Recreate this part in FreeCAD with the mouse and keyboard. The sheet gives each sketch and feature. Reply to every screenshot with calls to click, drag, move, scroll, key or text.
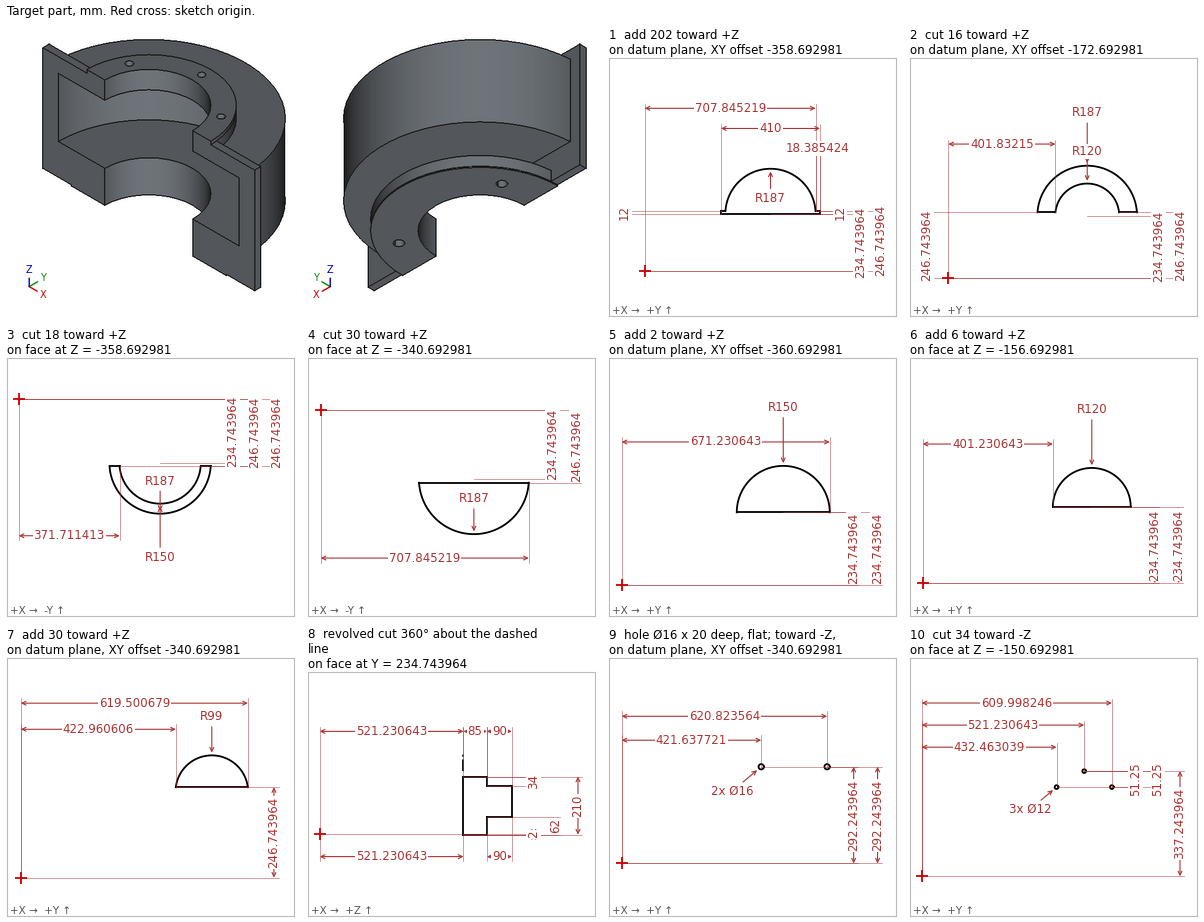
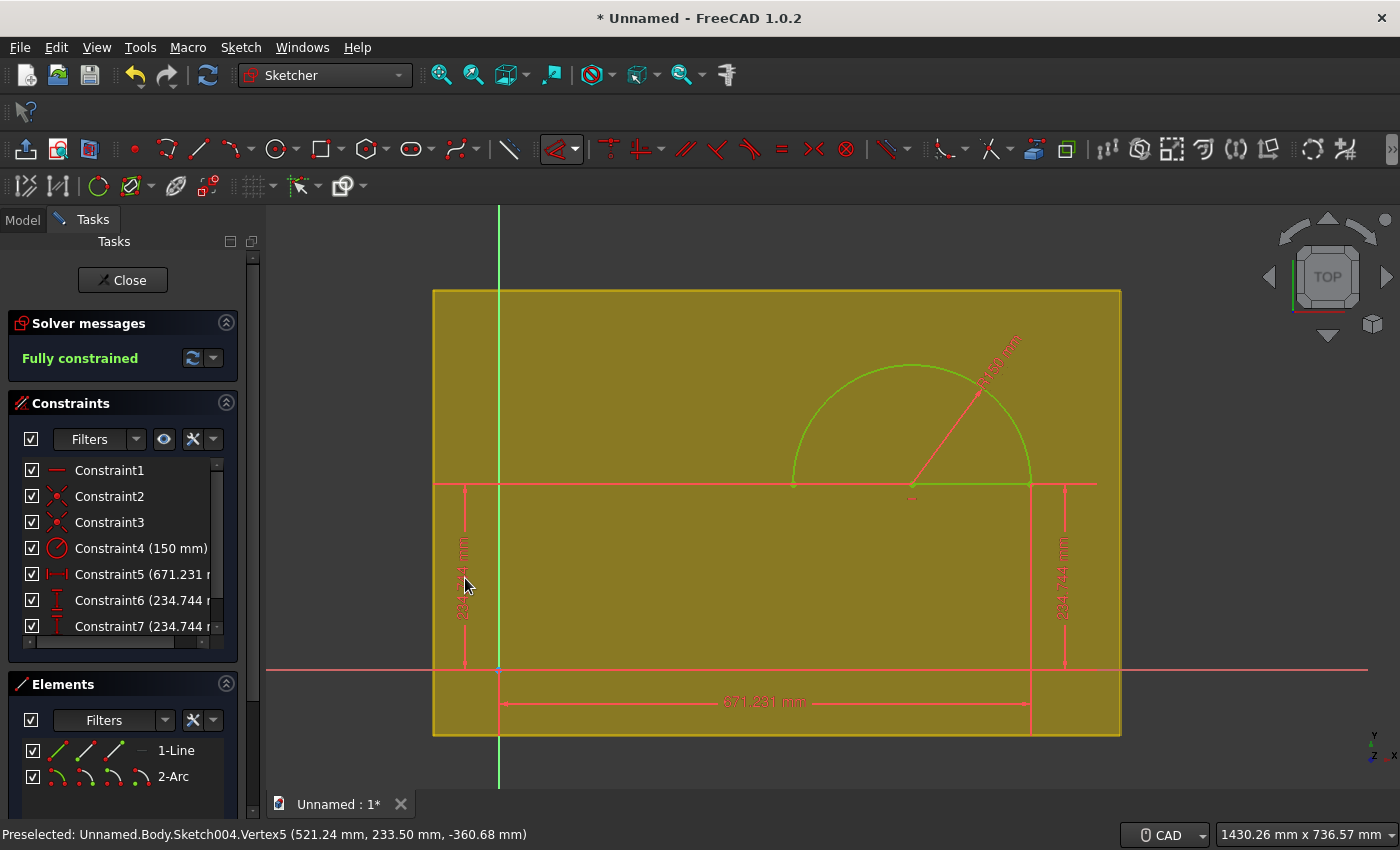
click(123, 280)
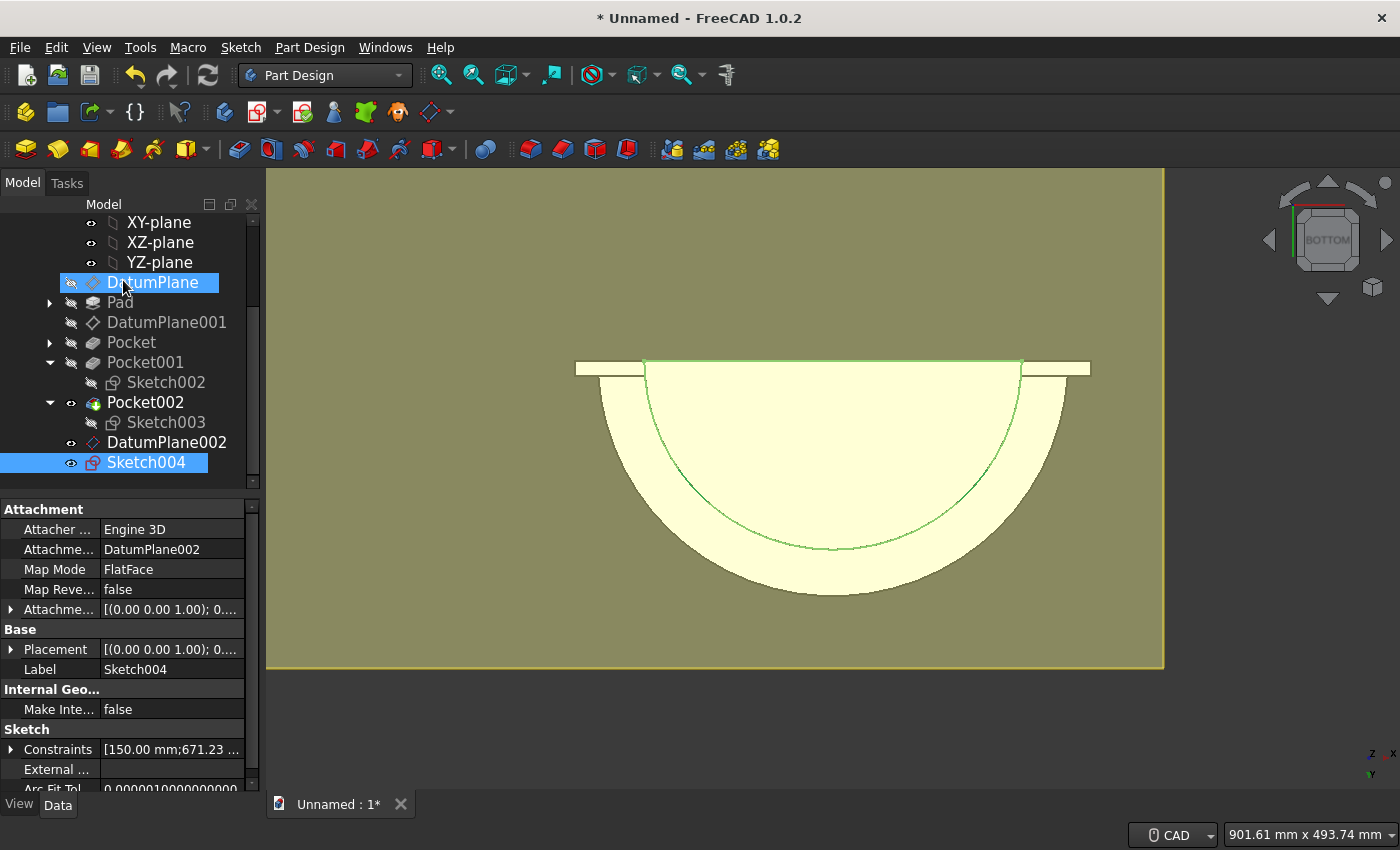
click(26, 150)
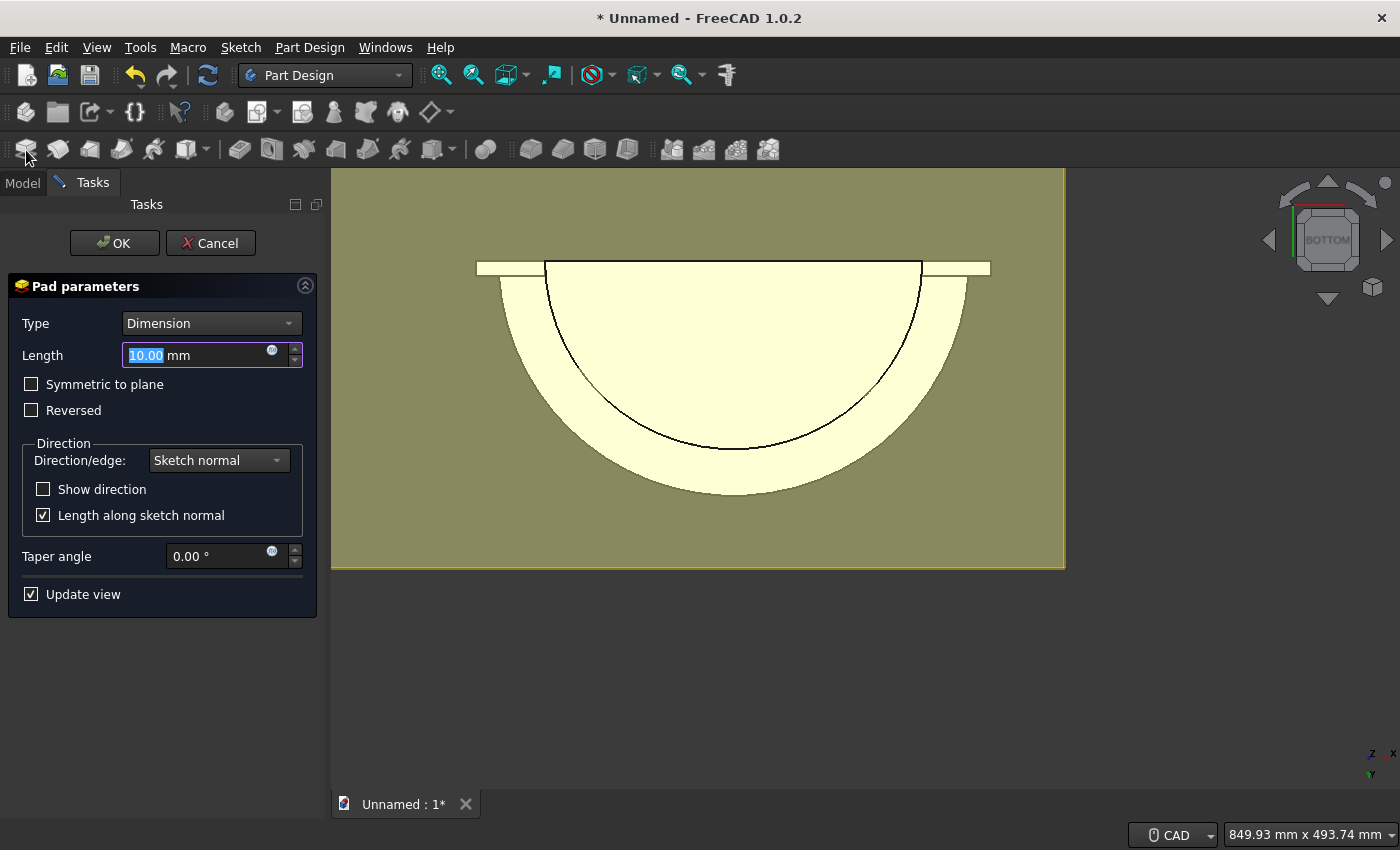
text(2)
key(Tab)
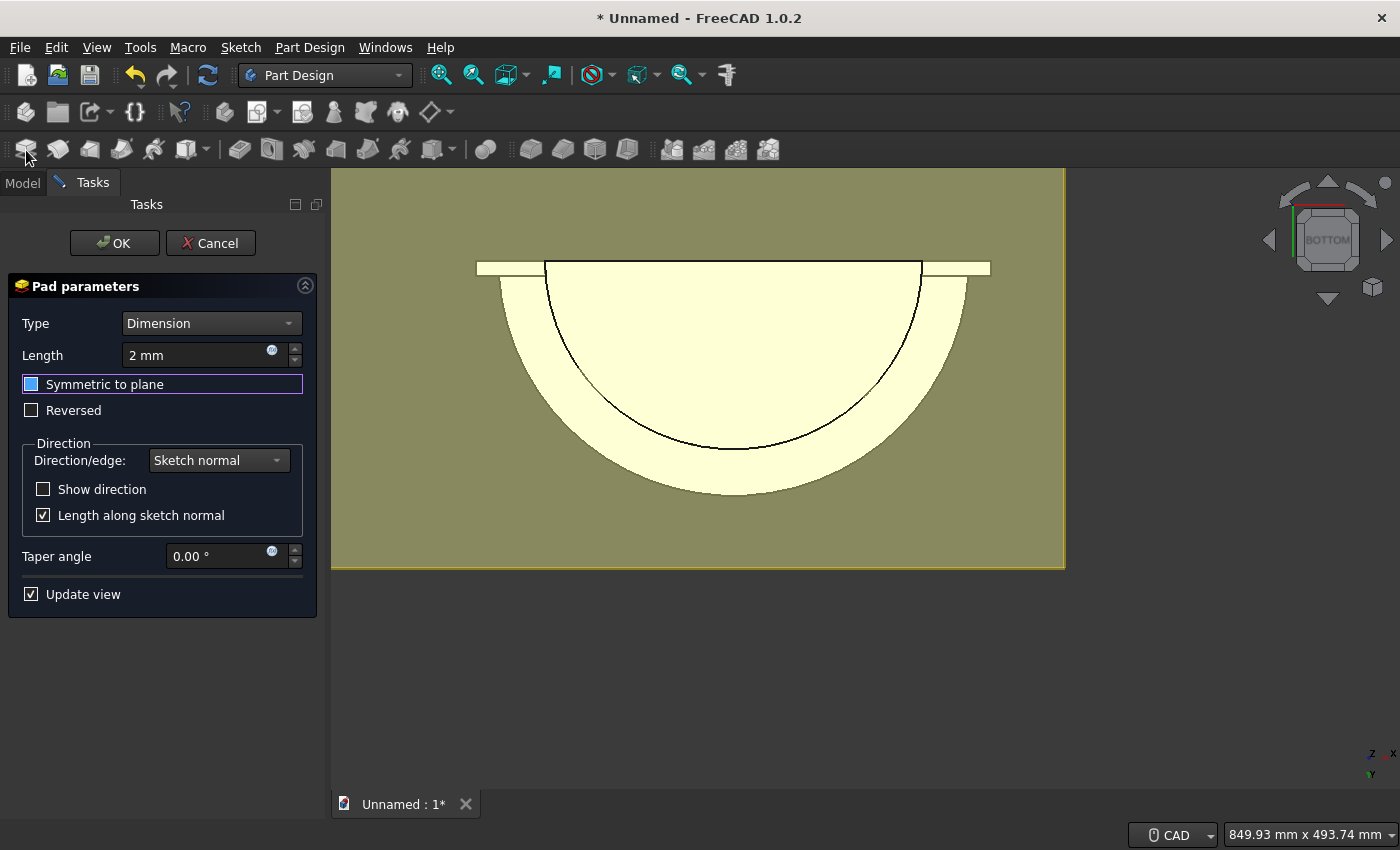
click(115, 243)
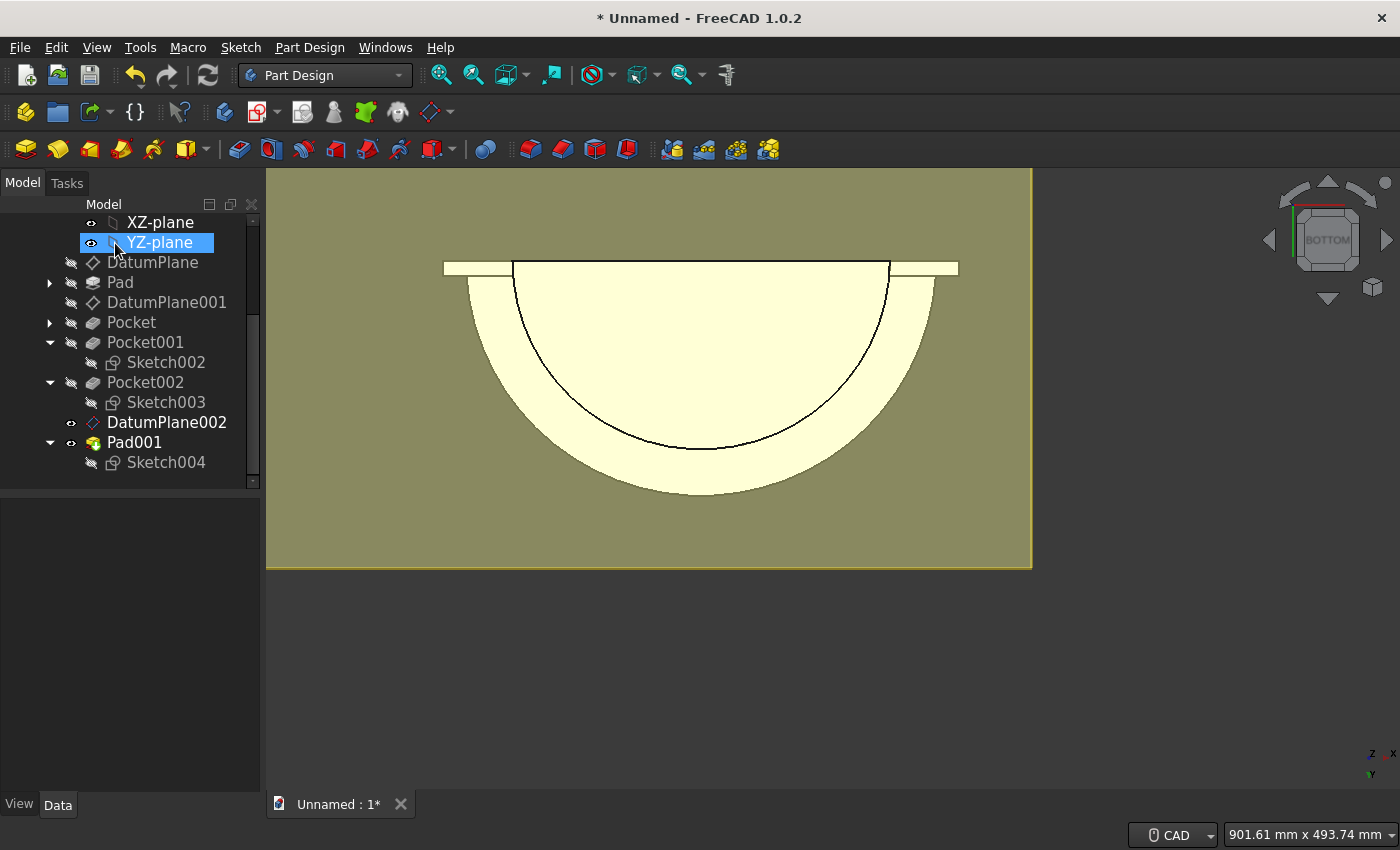
click(116, 423)
key(space)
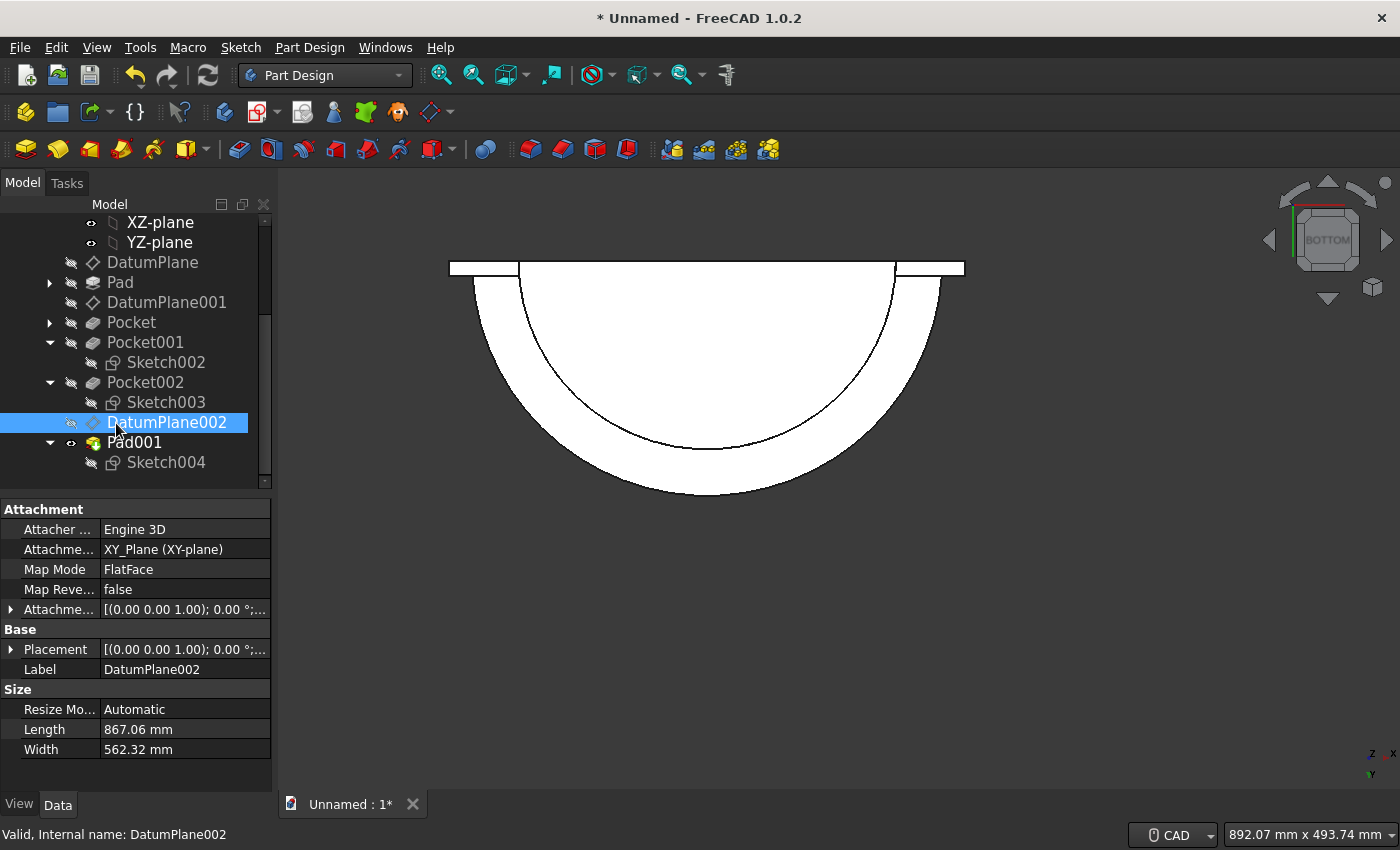
key(0)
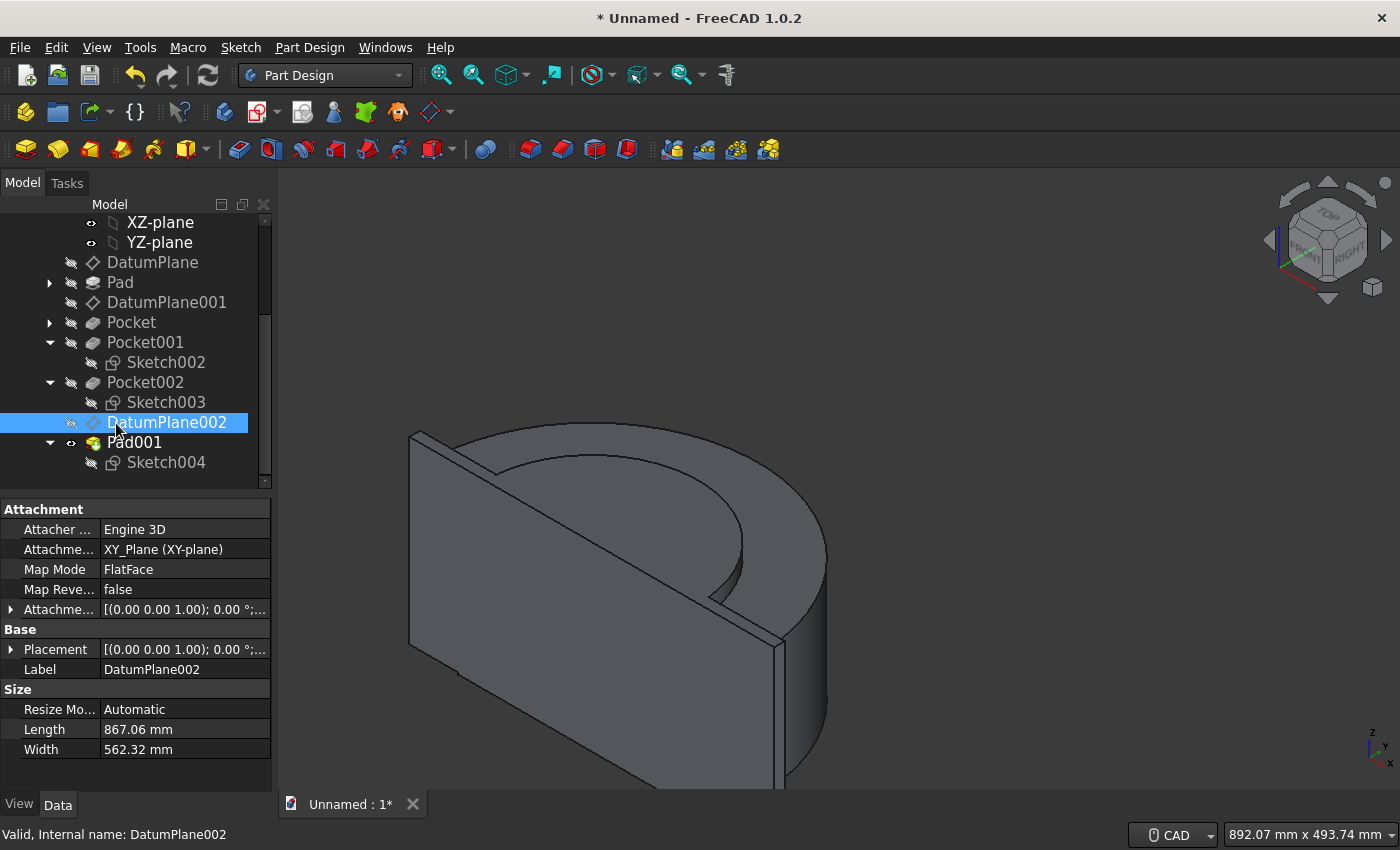
click(442, 76)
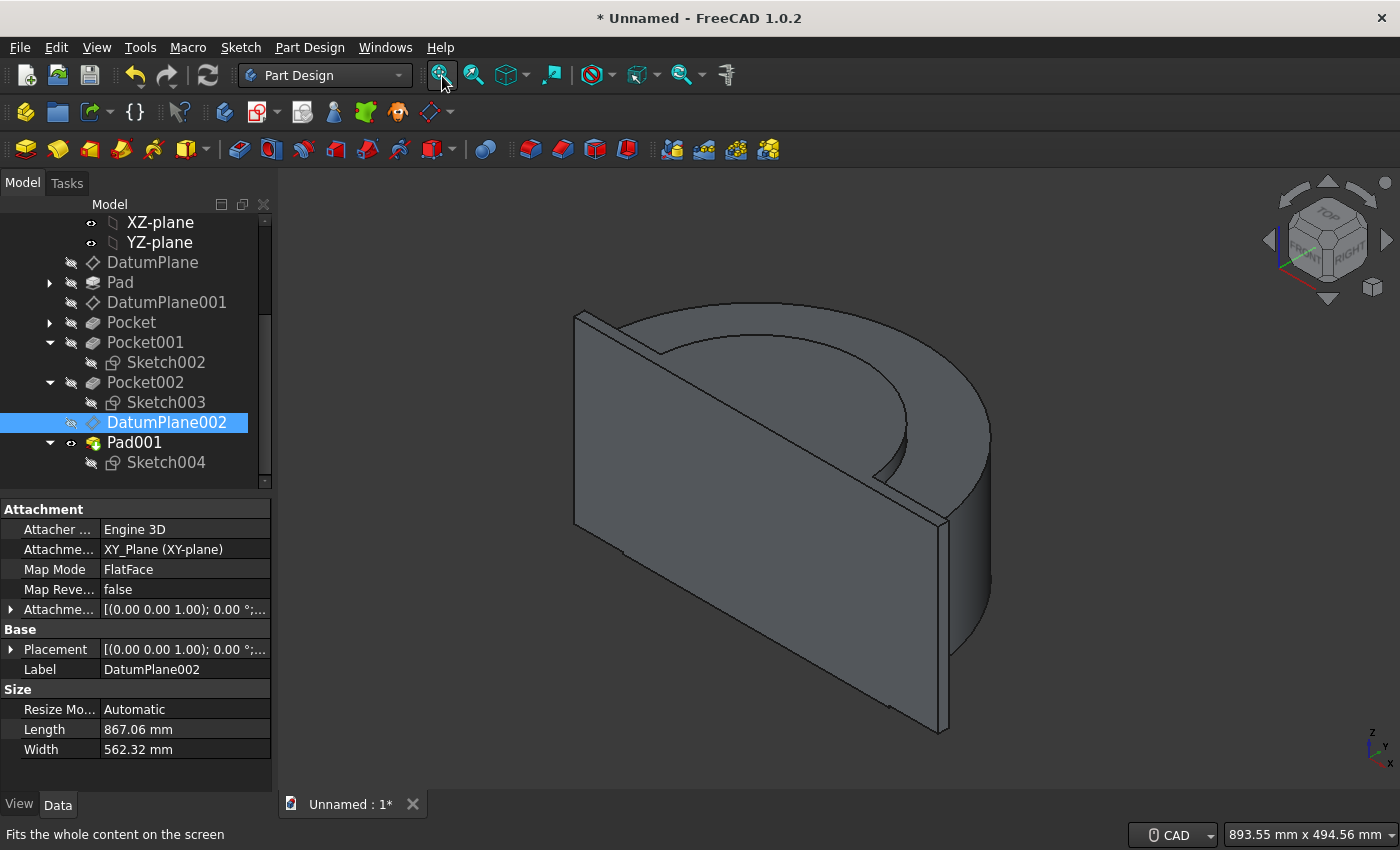
click(809, 390)